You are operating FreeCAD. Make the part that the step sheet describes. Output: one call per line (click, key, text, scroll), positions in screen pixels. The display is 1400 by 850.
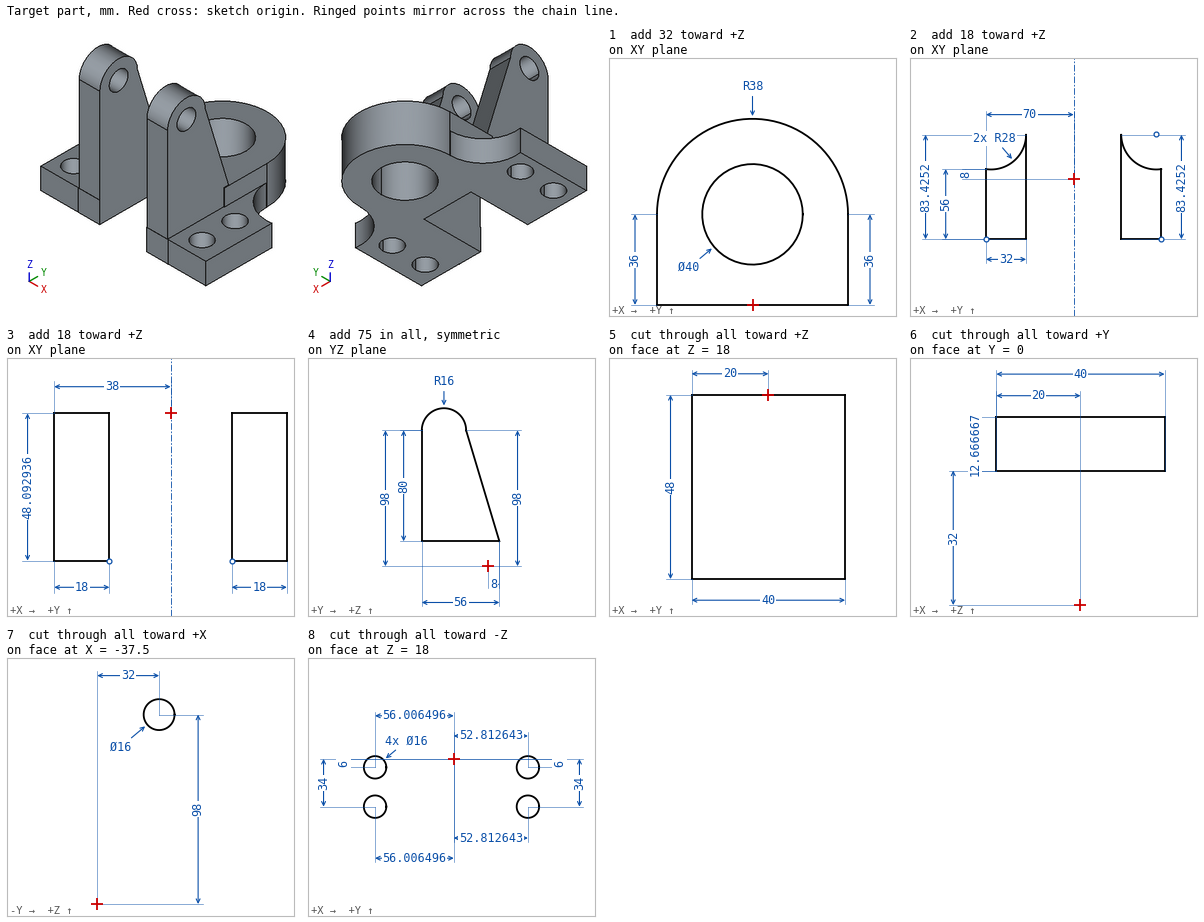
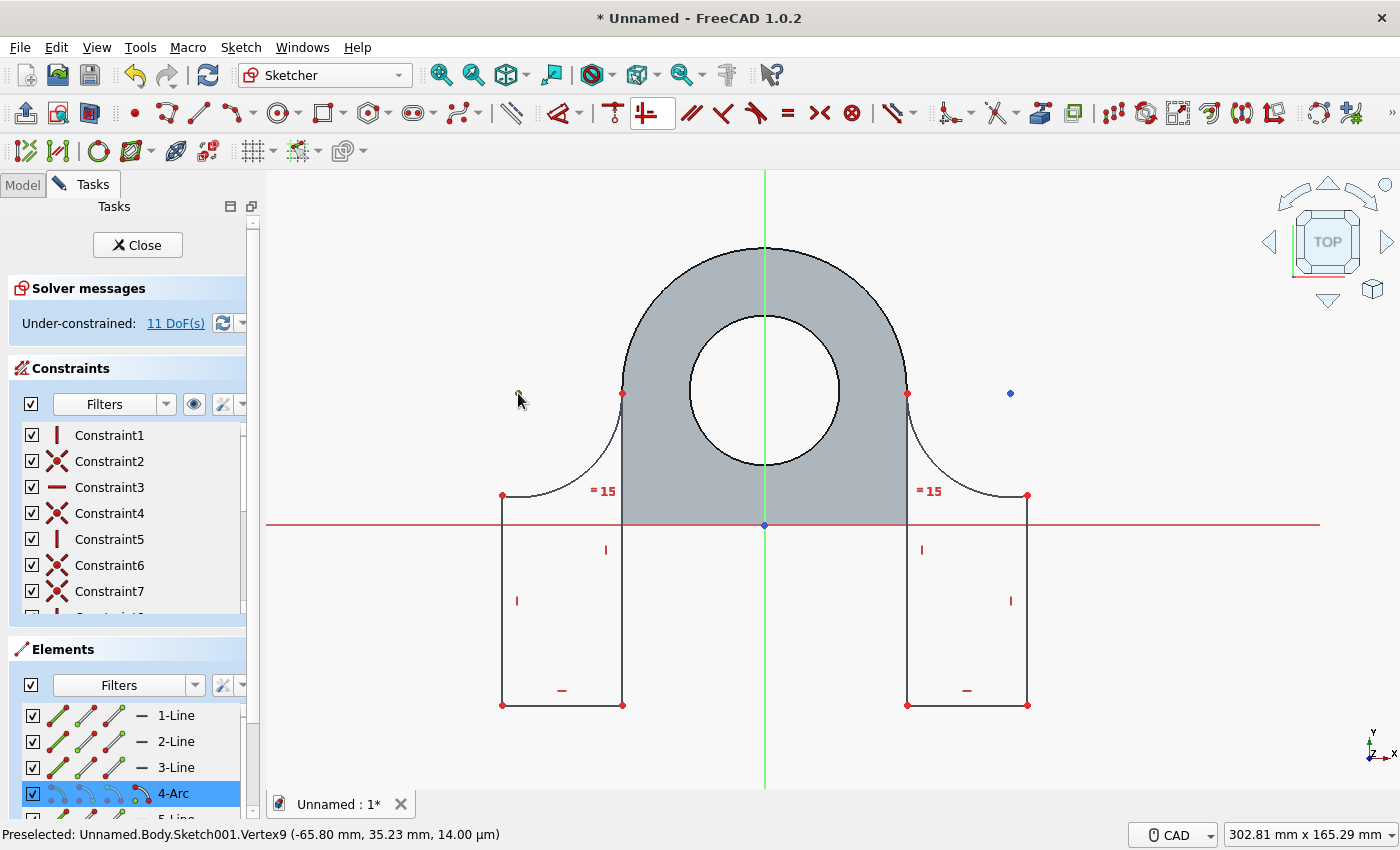
click(1011, 393)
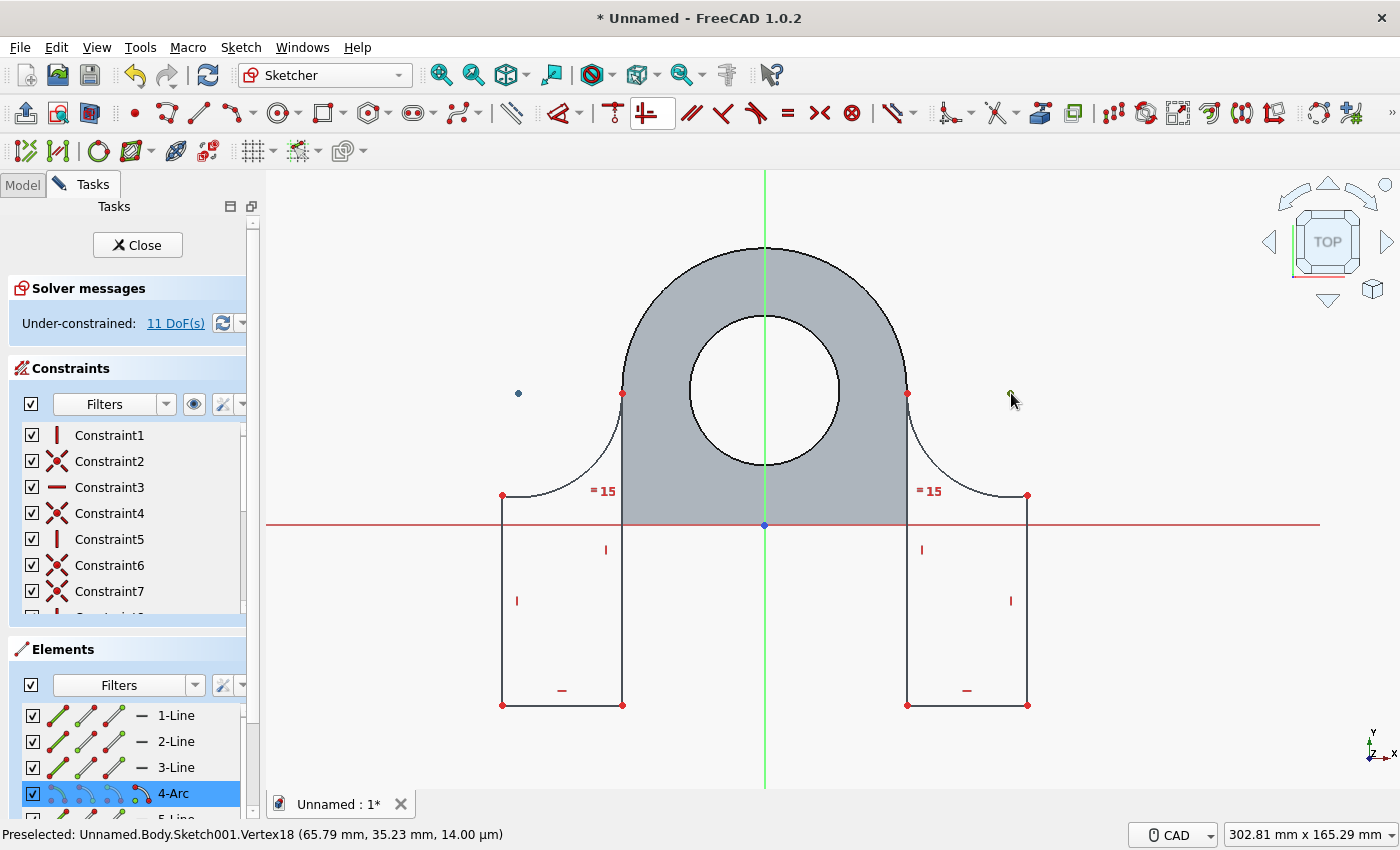
click(765, 721)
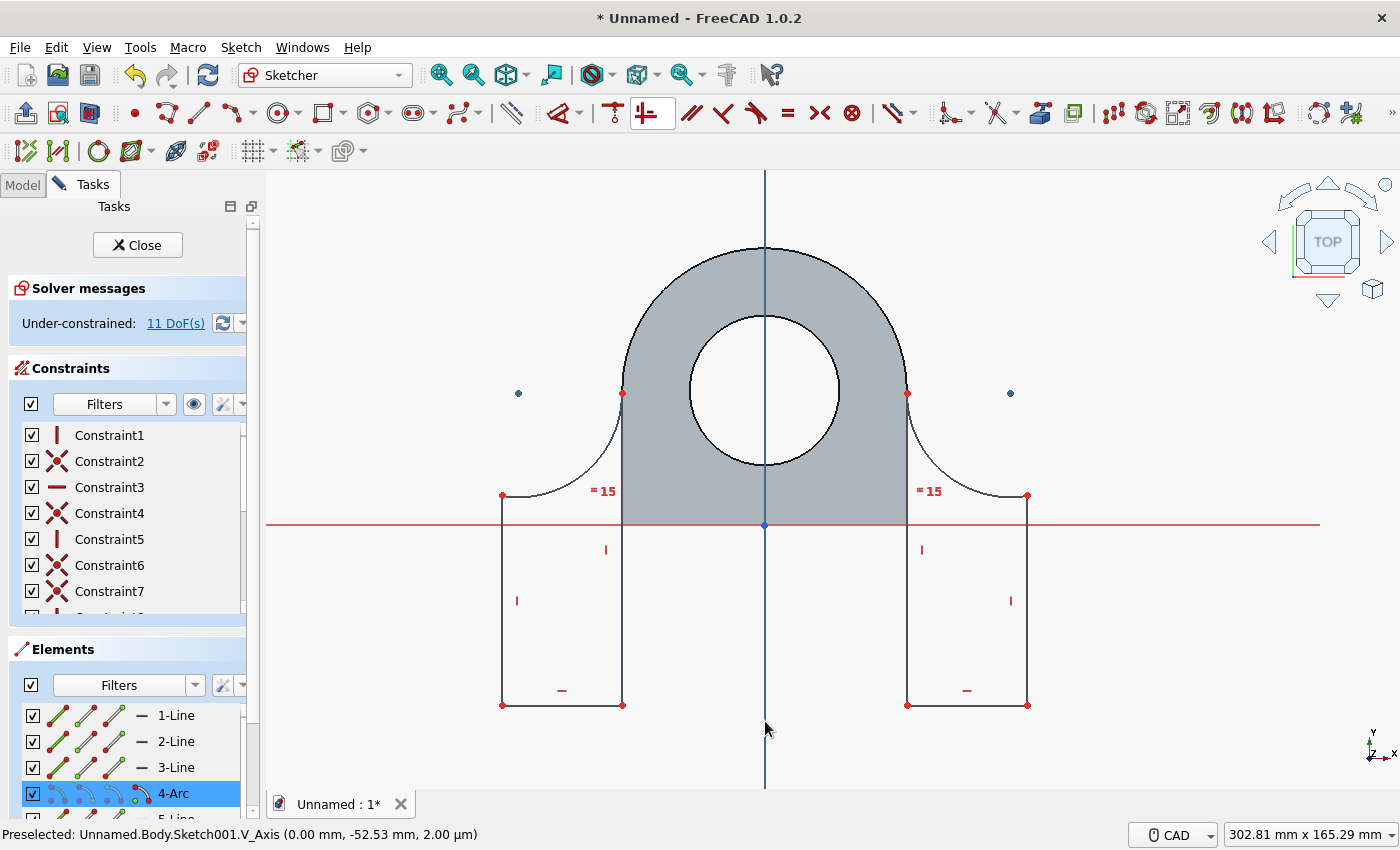
click(820, 114)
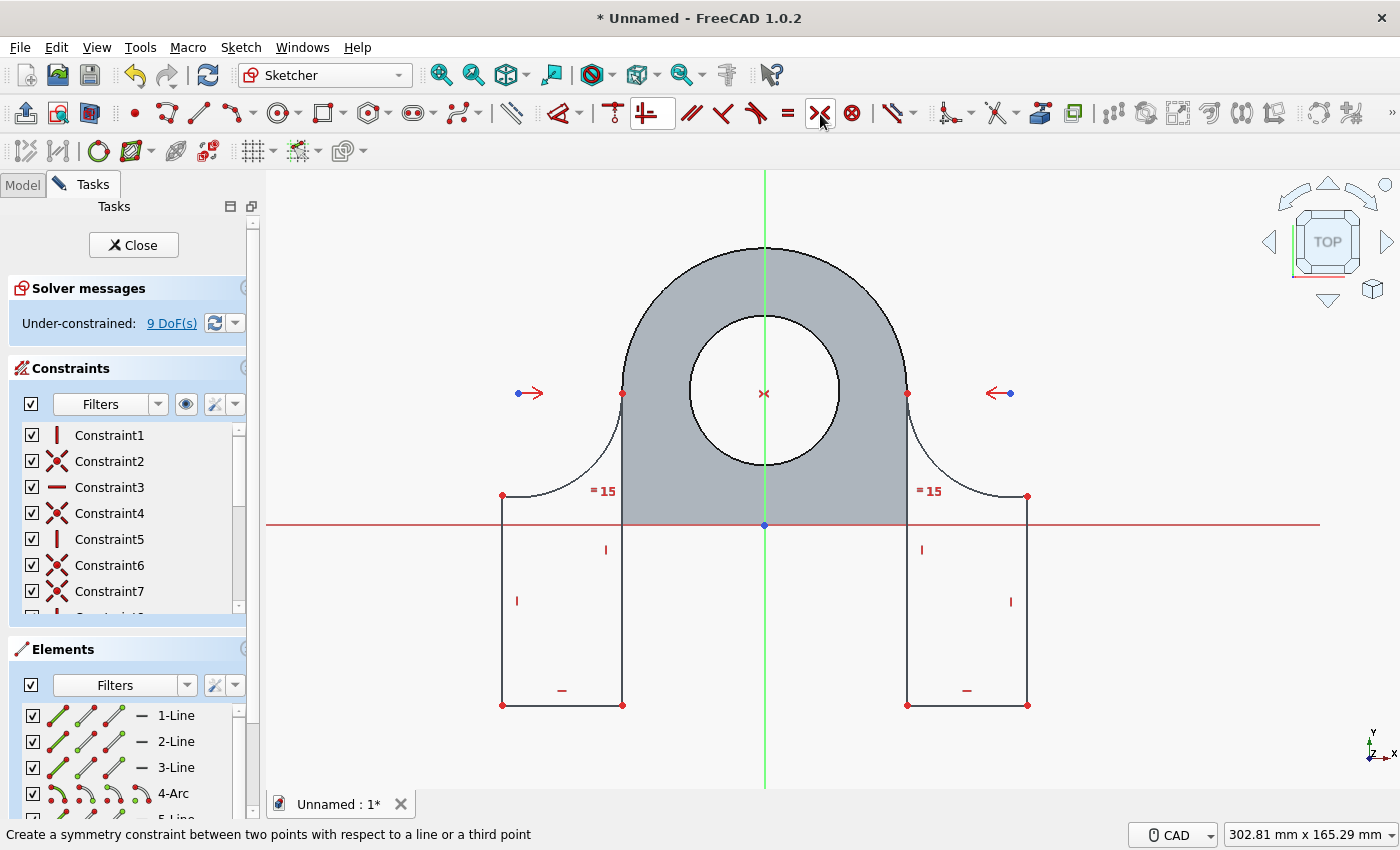
click(502, 706)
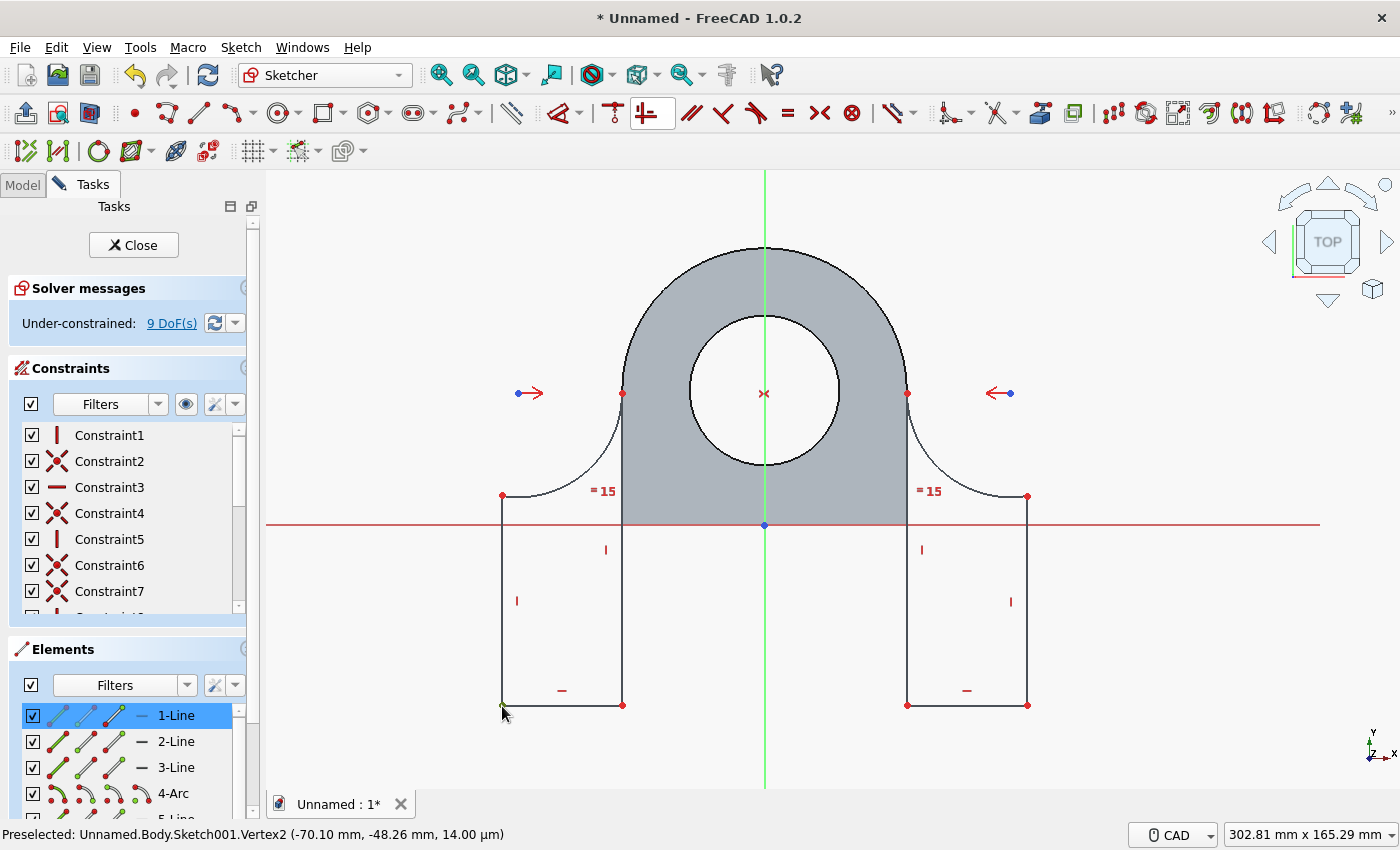
click(1027, 706)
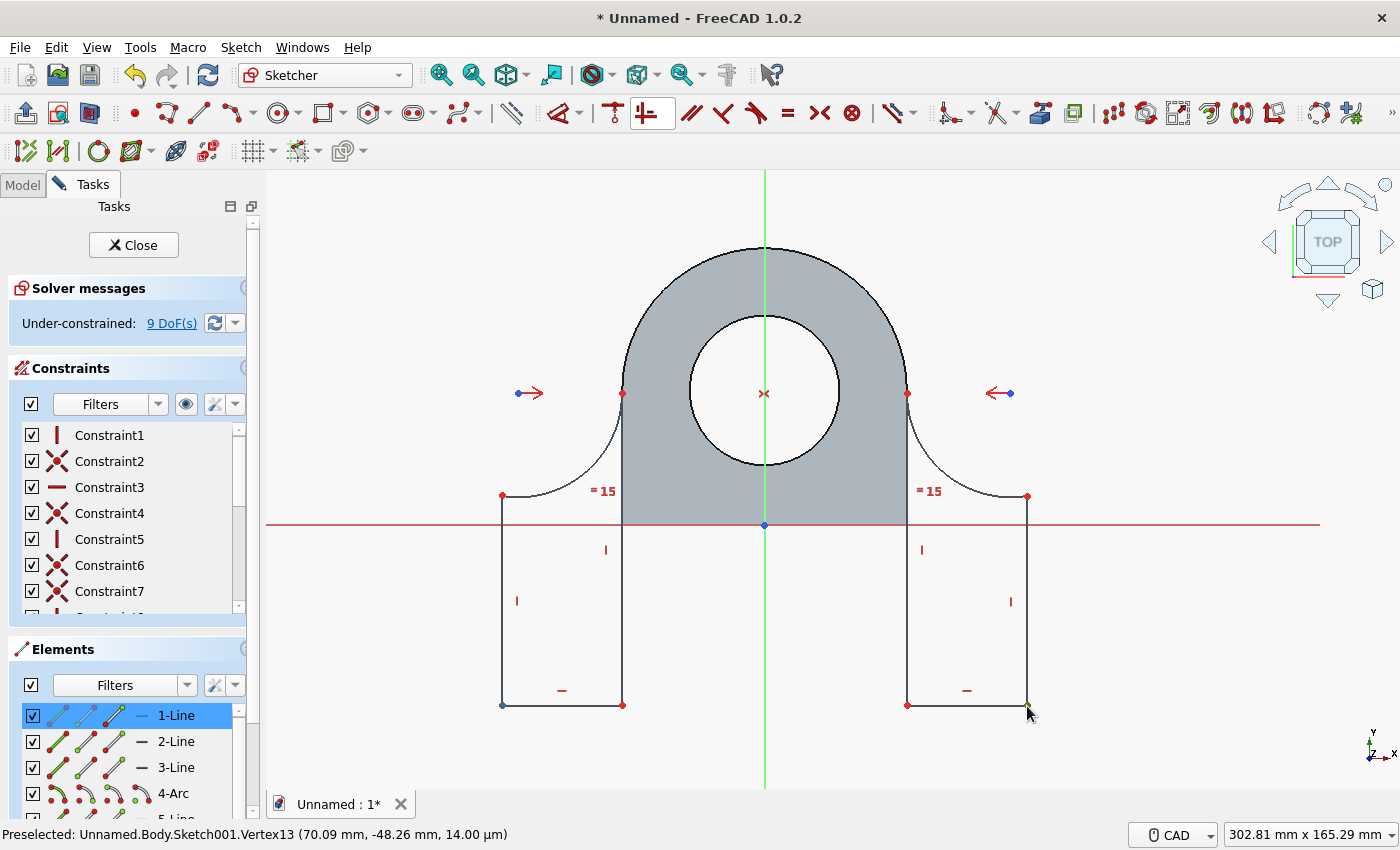
click(765, 721)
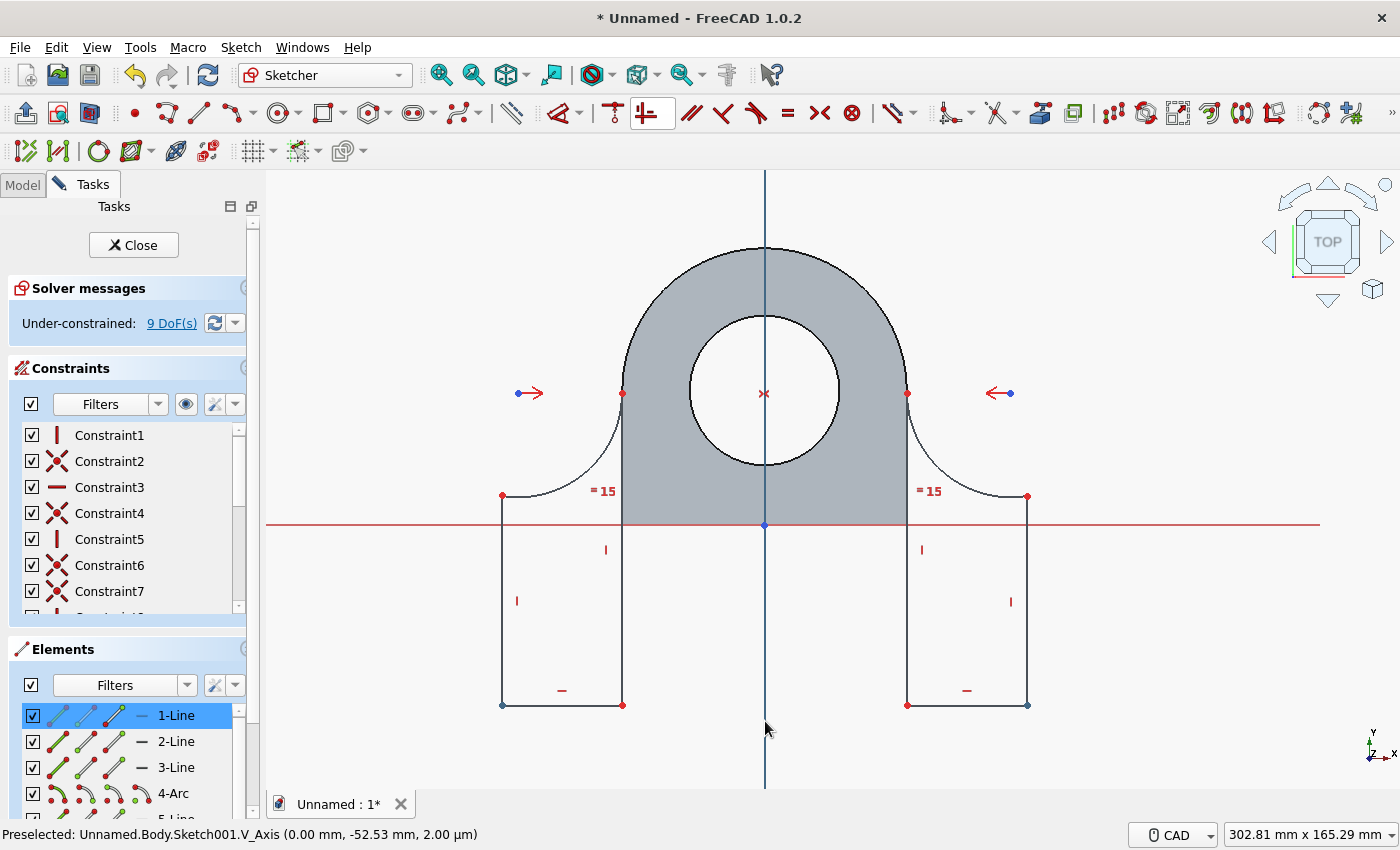
click(820, 114)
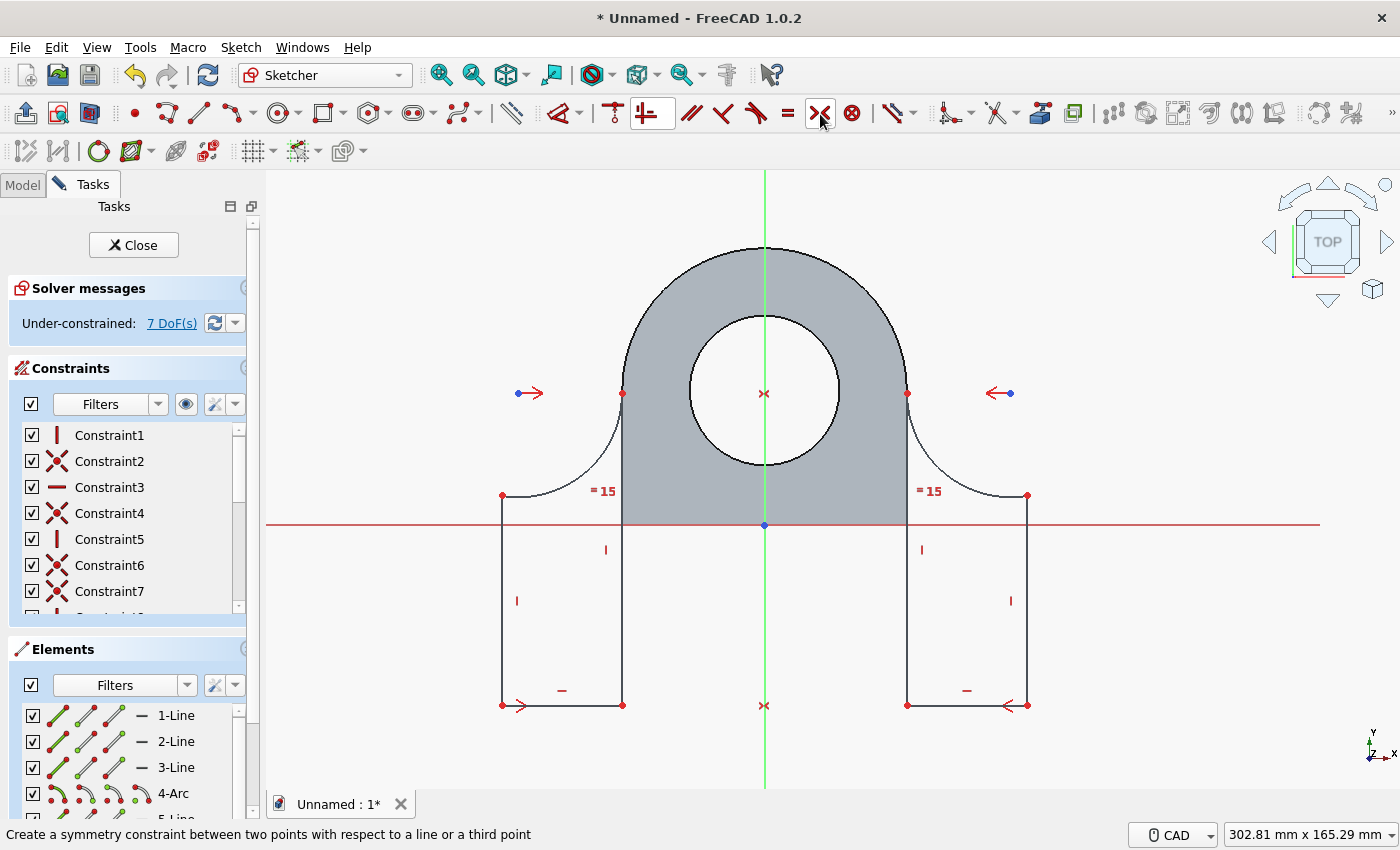
click(558, 114)